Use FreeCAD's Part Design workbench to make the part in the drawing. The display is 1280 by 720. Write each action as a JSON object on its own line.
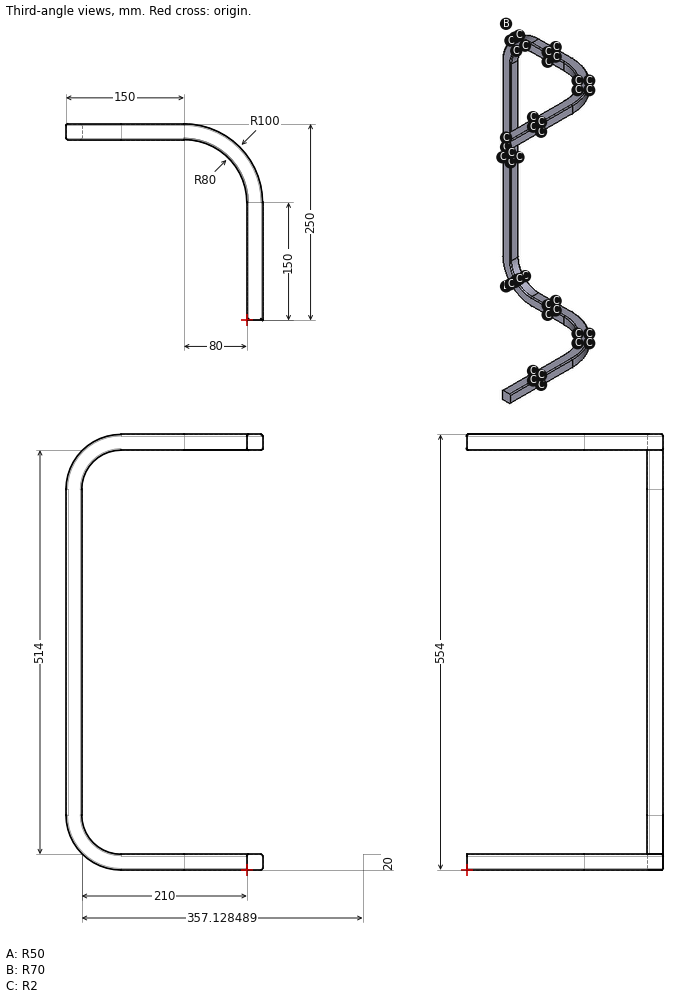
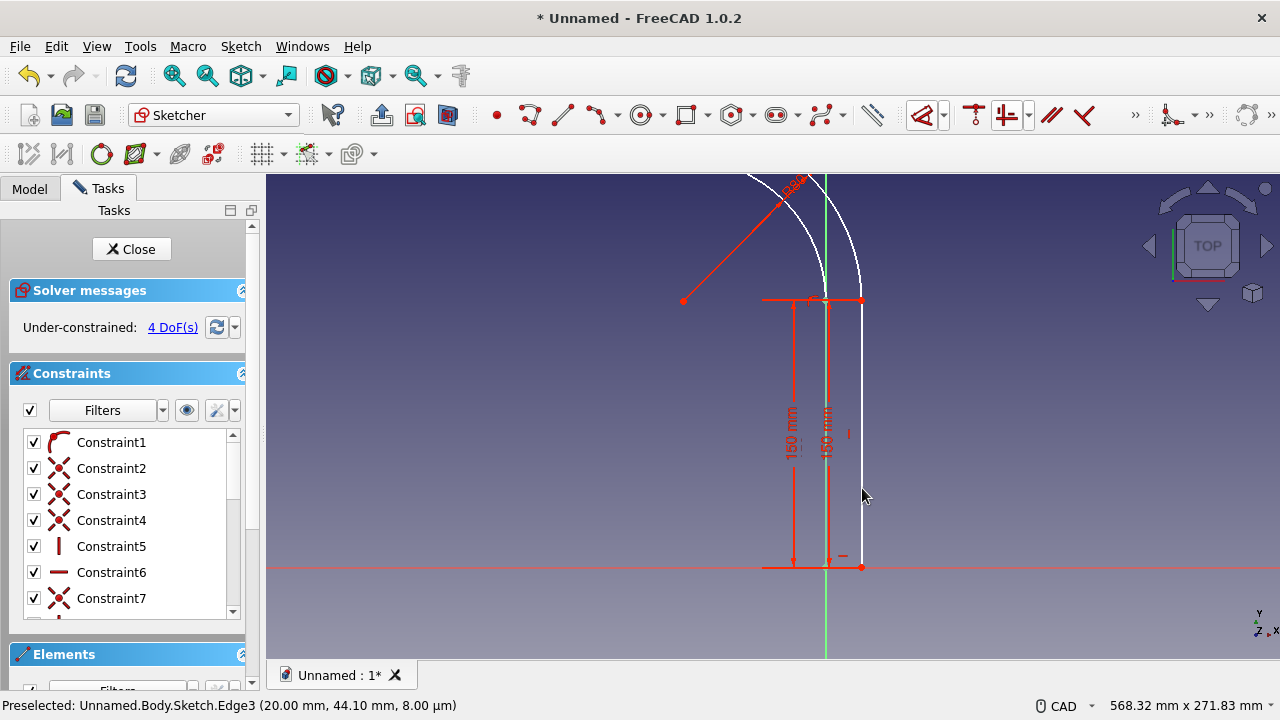
{"action": "scroll", "coordinate": [839, 563], "scroll_direction": "down", "scroll_amount": 2}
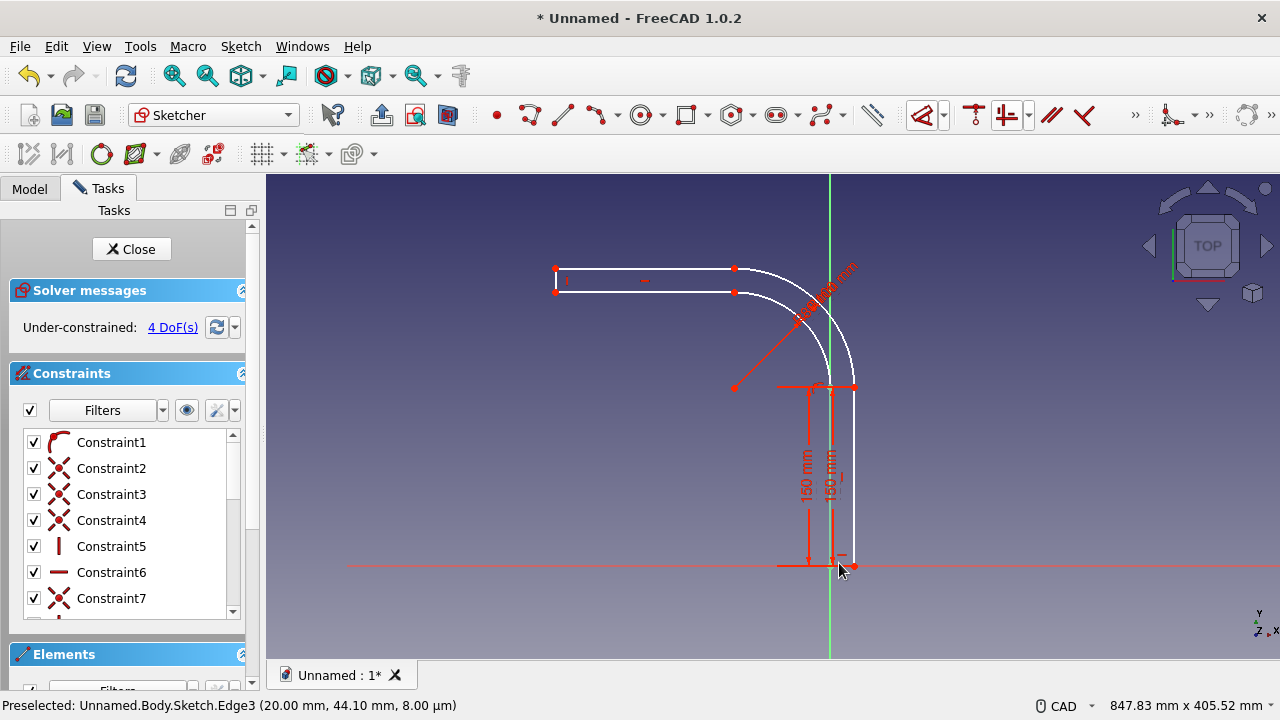
{"action": "left_click", "coordinate": [681, 269]}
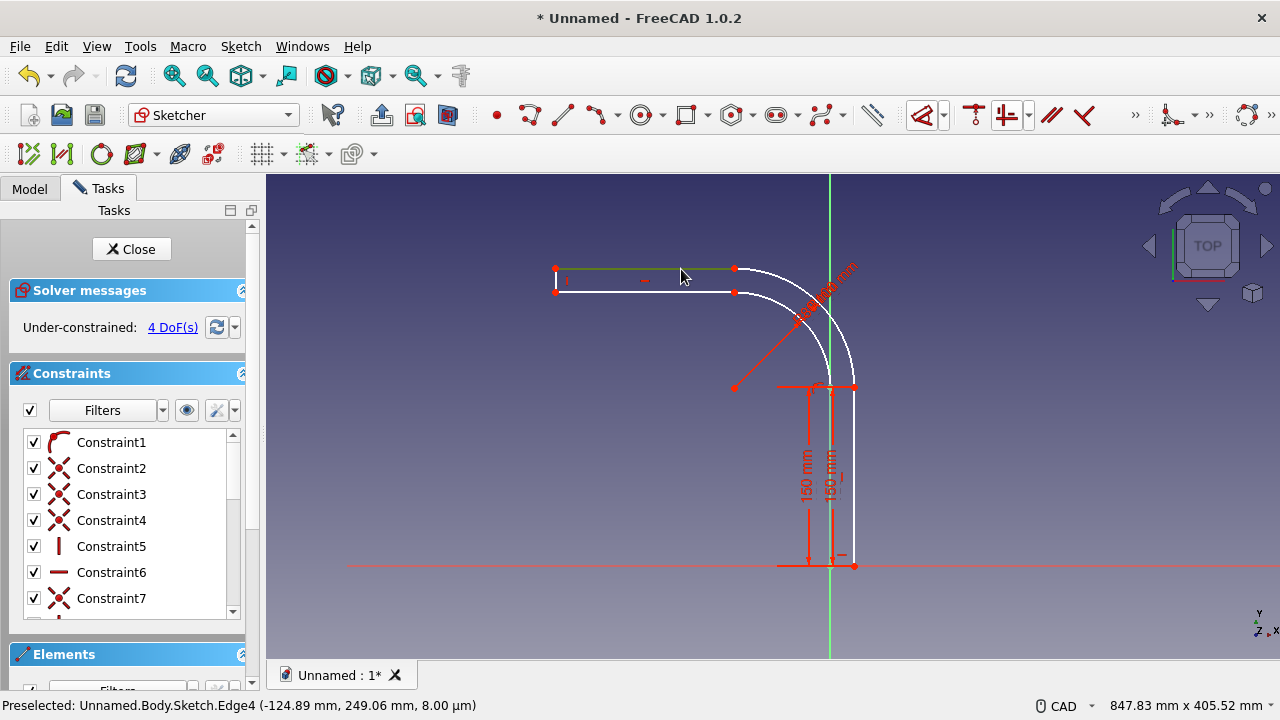
{"action": "left_click", "coordinate": [944, 116]}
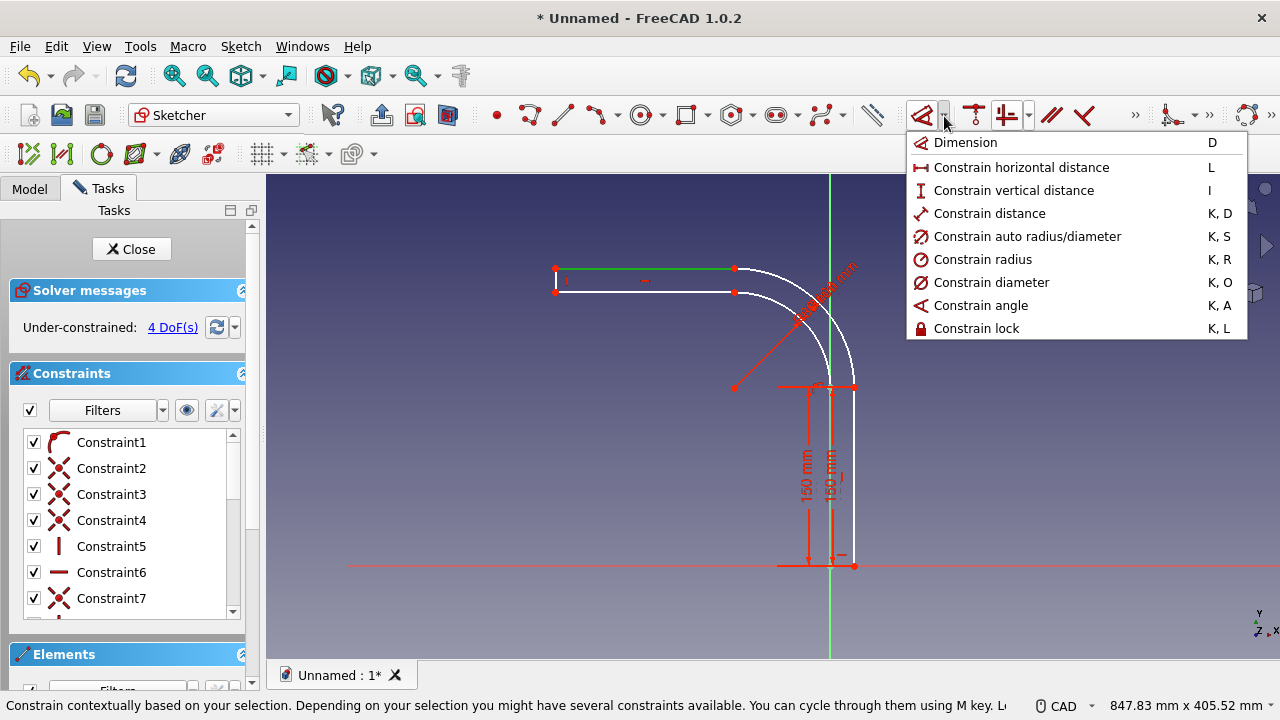
{"action": "left_click", "coordinate": [1077, 168]}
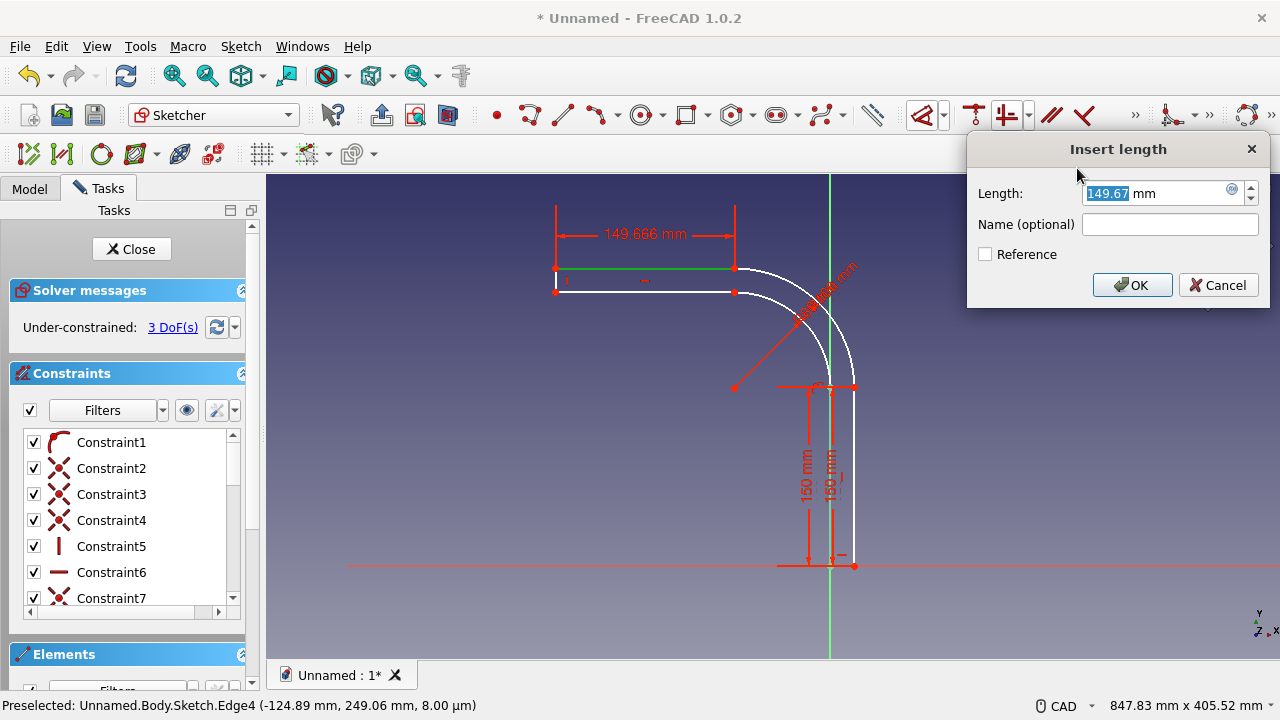
{"action": "type", "text": "150"}
{"action": "key", "text": "Return"}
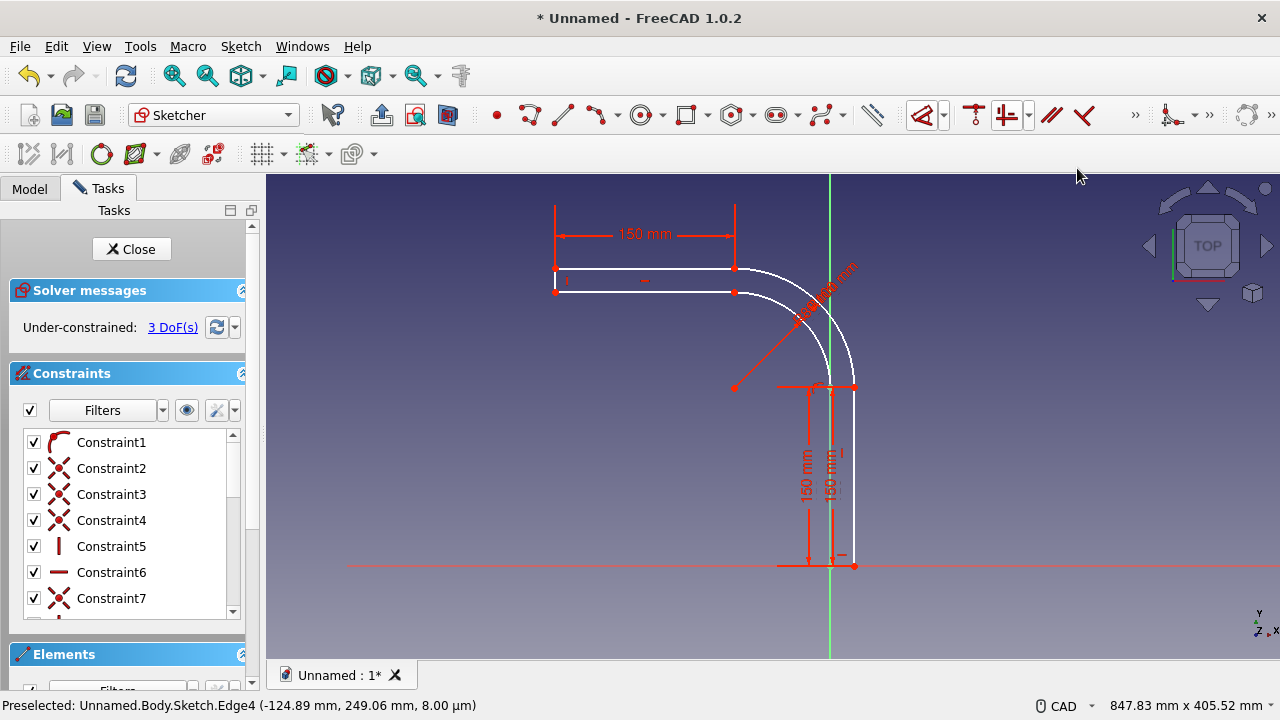
{"action": "left_click", "coordinate": [609, 292]}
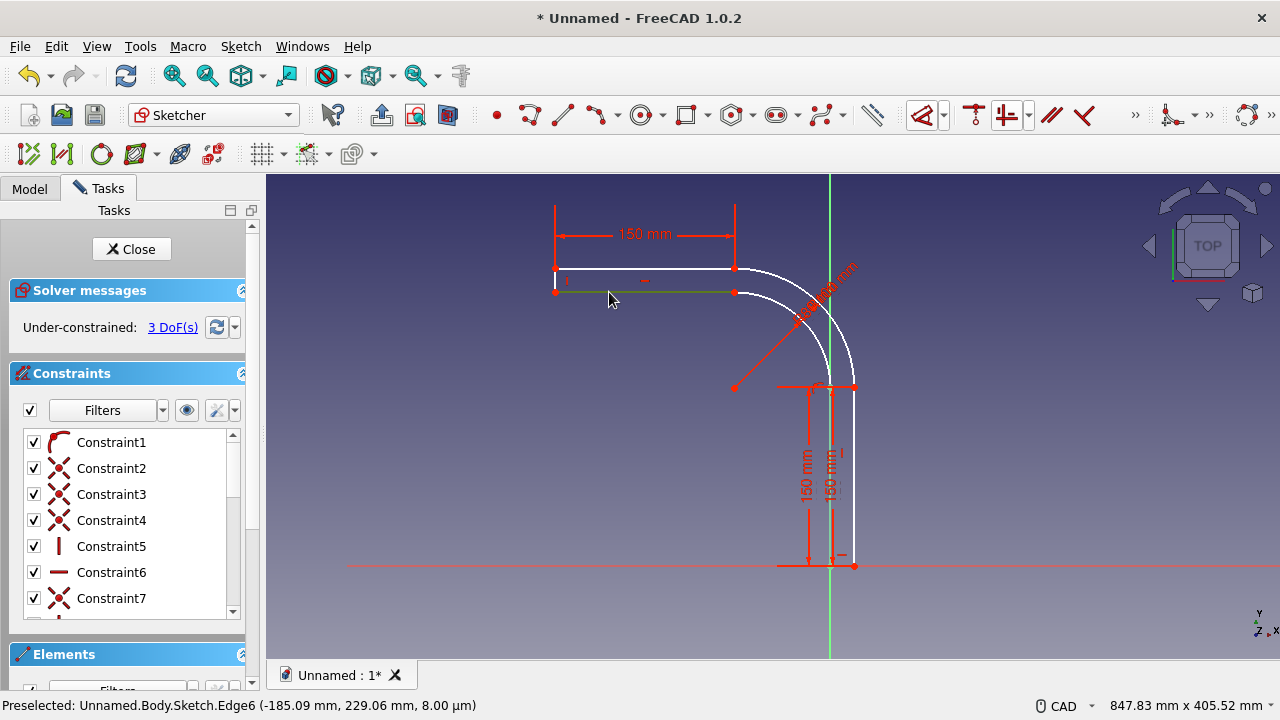
{"action": "key", "text": "l"}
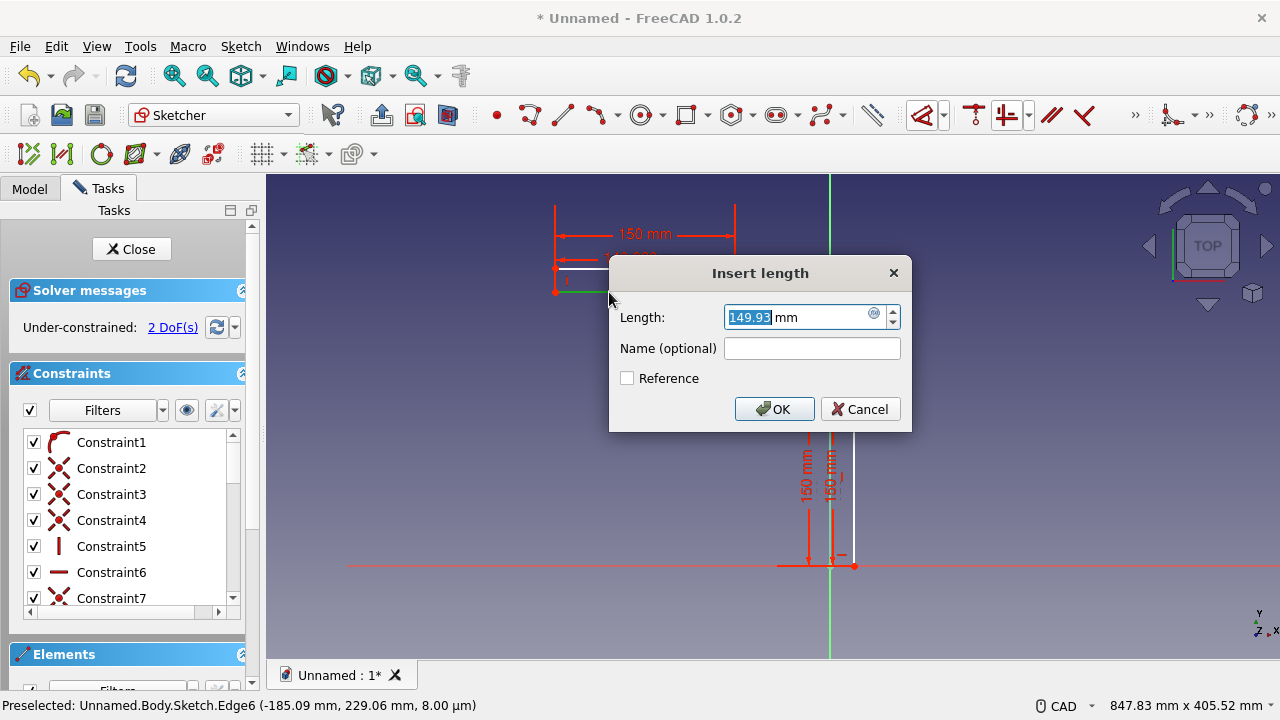
{"action": "type", "text": "150"}
{"action": "key", "text": "Return"}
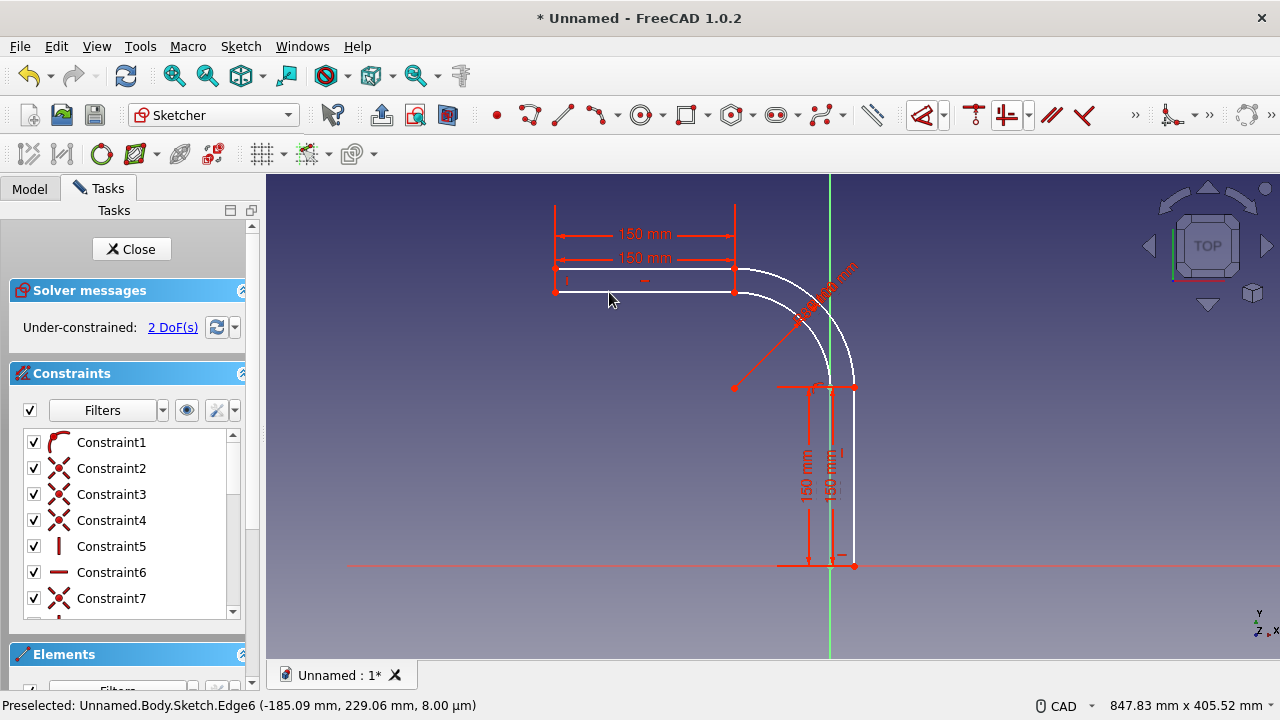
{"action": "left_click", "coordinate": [735, 269]}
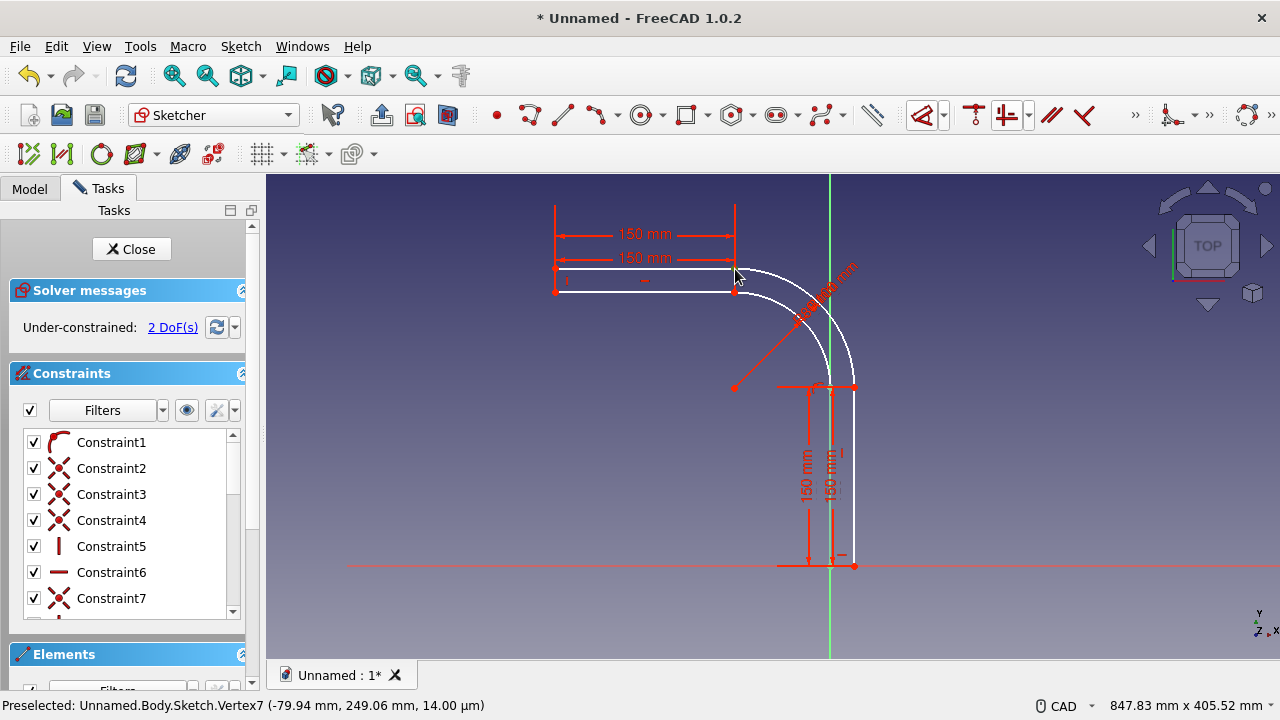
{"action": "left_click", "coordinate": [944, 116]}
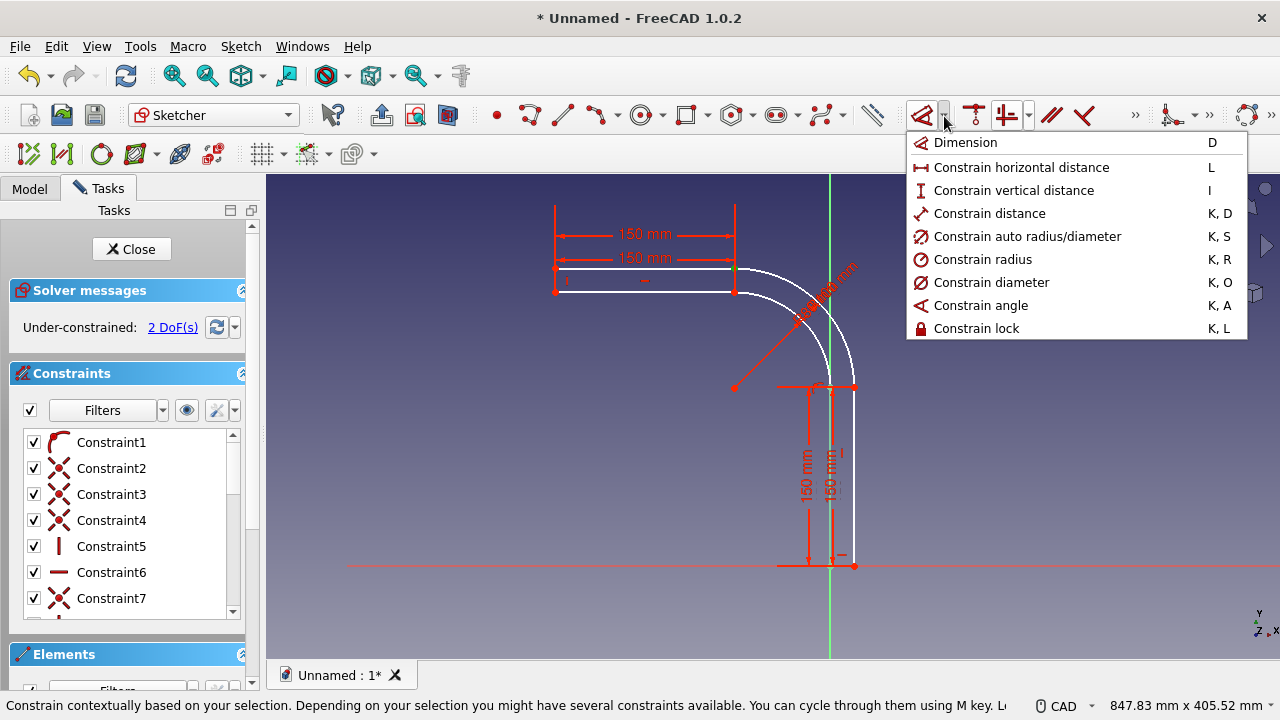
{"action": "left_click", "coordinate": [1077, 168]}